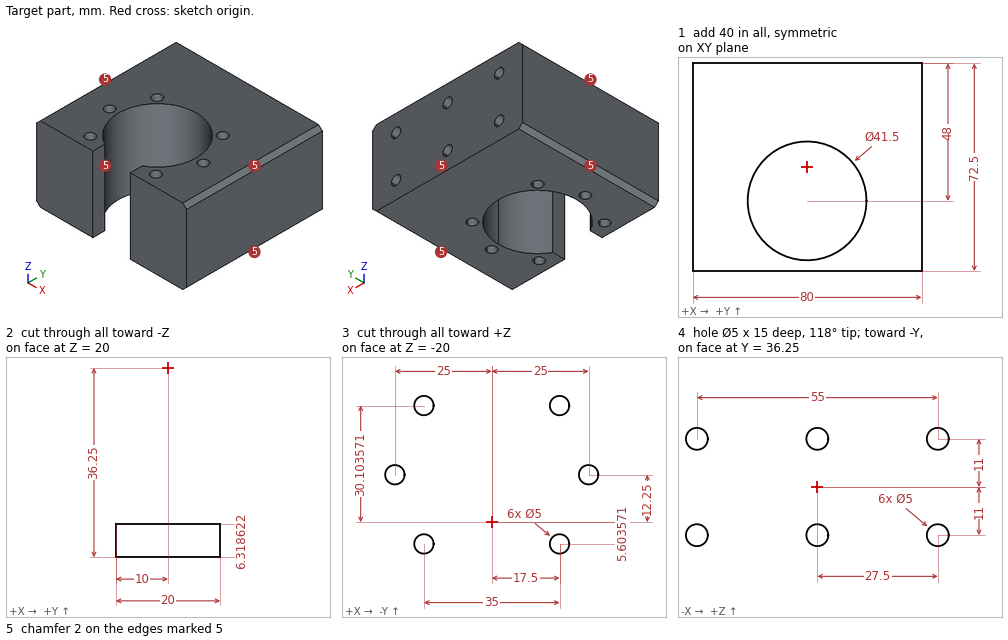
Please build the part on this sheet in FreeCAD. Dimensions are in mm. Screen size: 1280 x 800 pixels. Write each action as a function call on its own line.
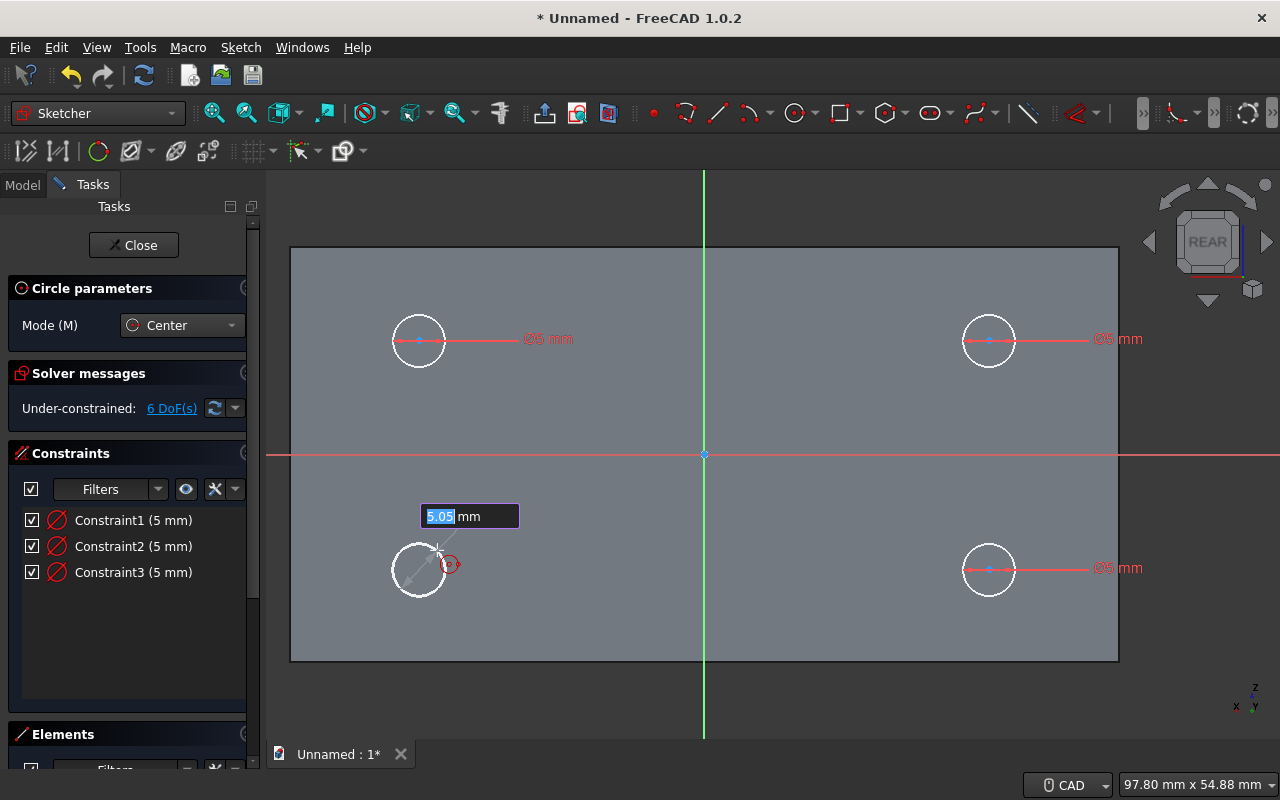
text(5)
key(Return)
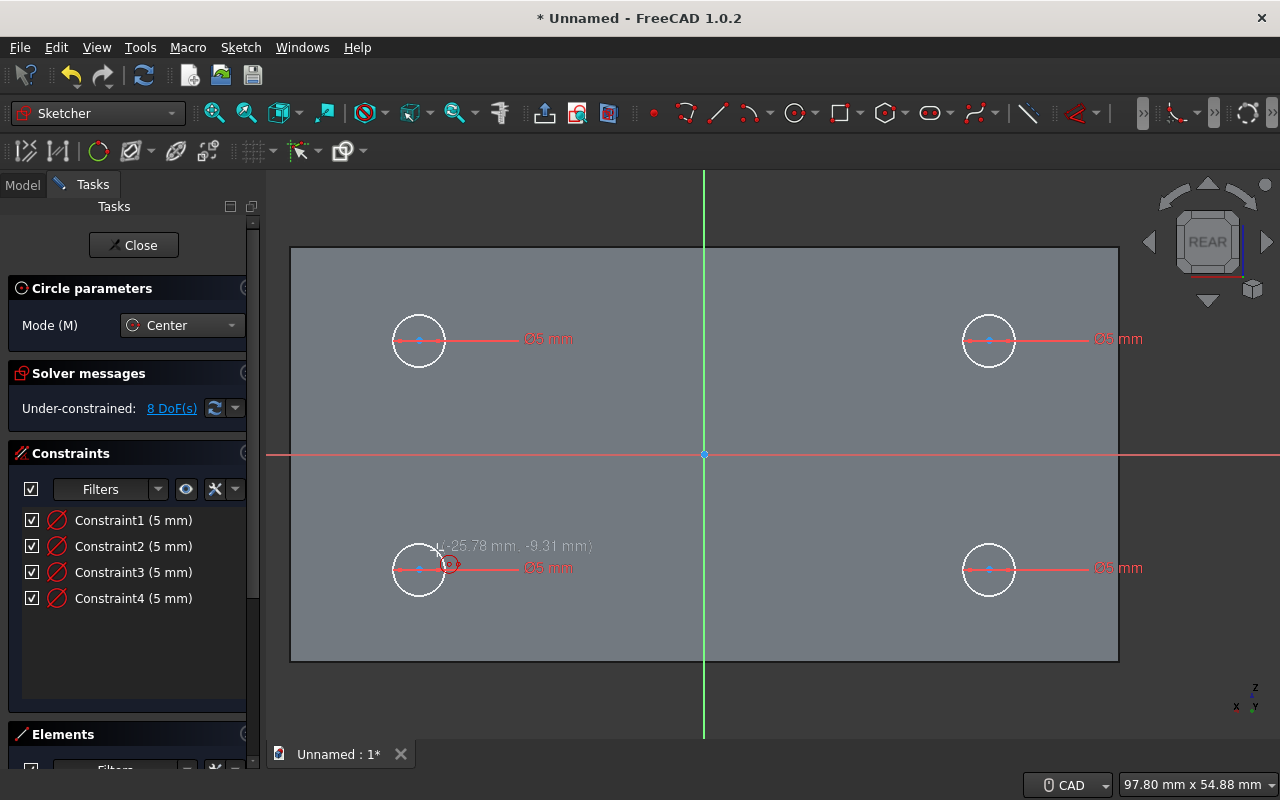
click(704, 569)
move(723, 550)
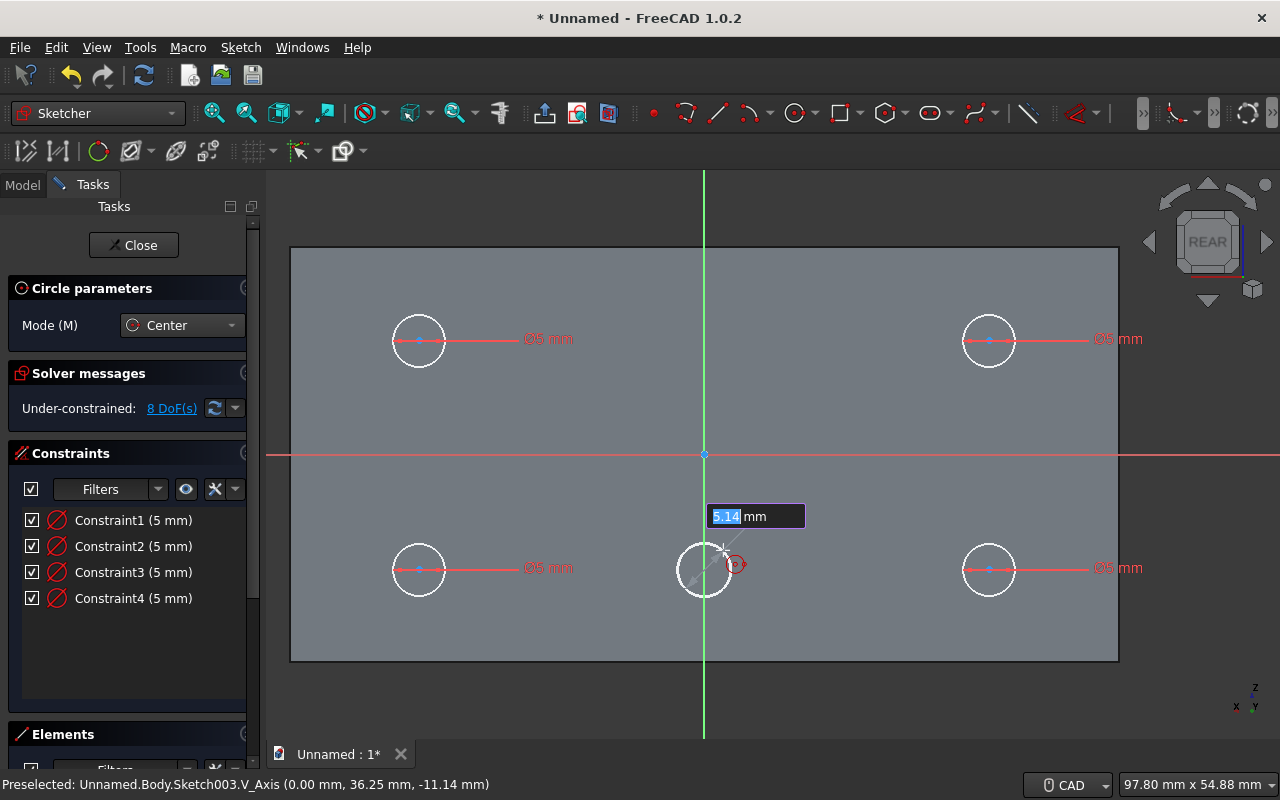
text(5)
key(Return)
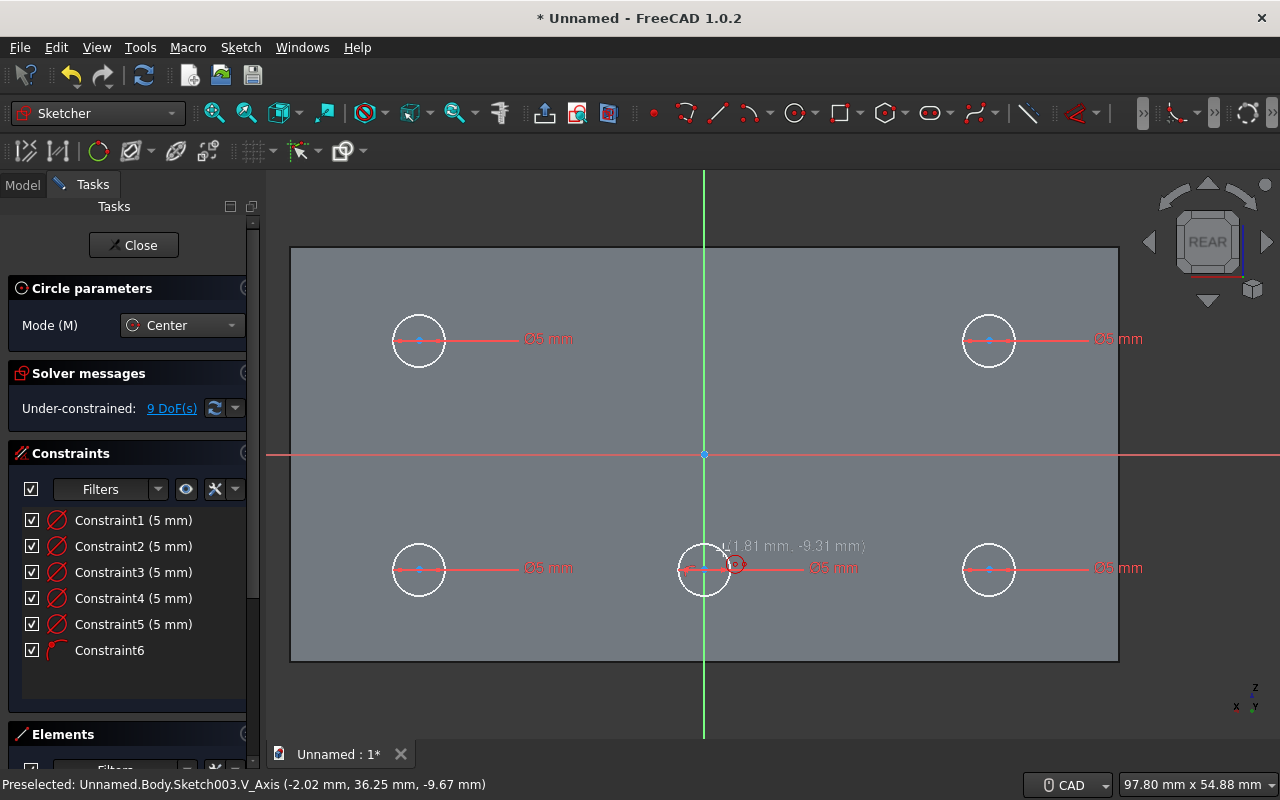
click(704, 340)
move(723, 322)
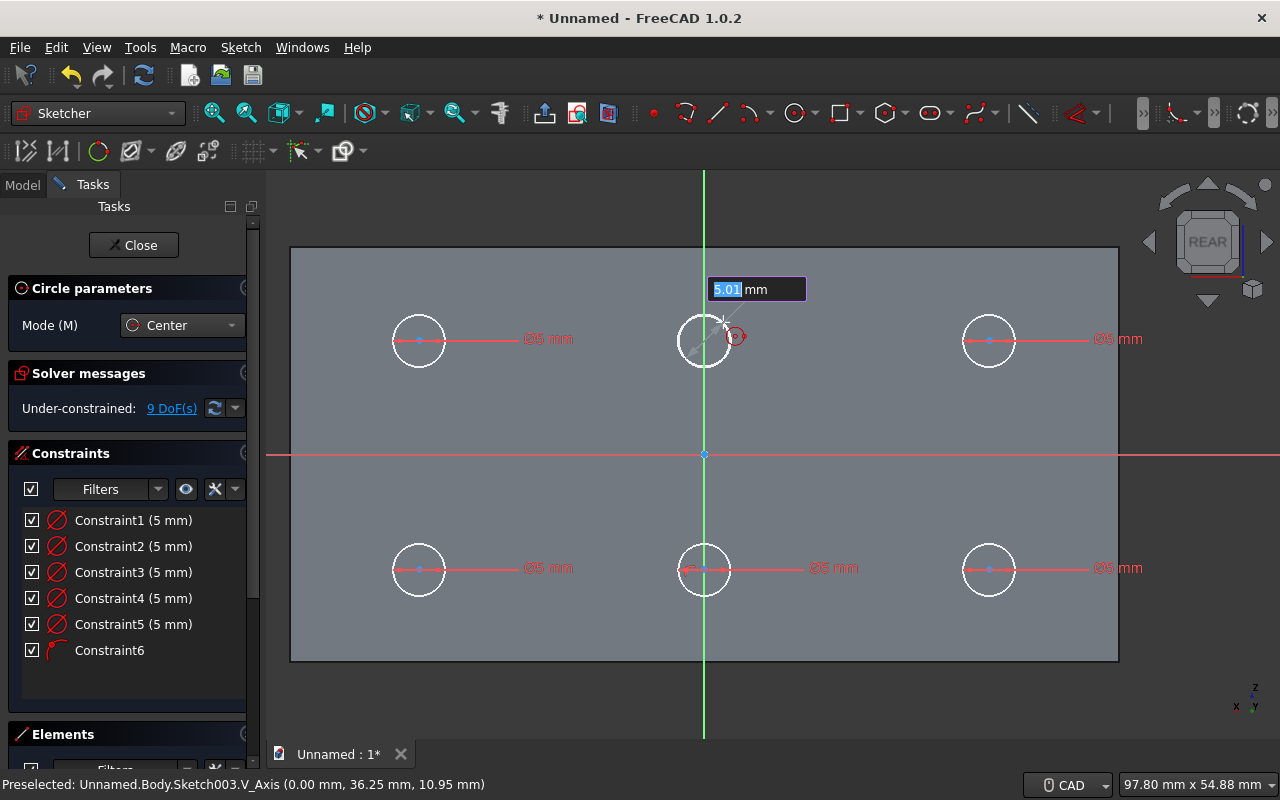
text(5)
key(Return)
key(Escape)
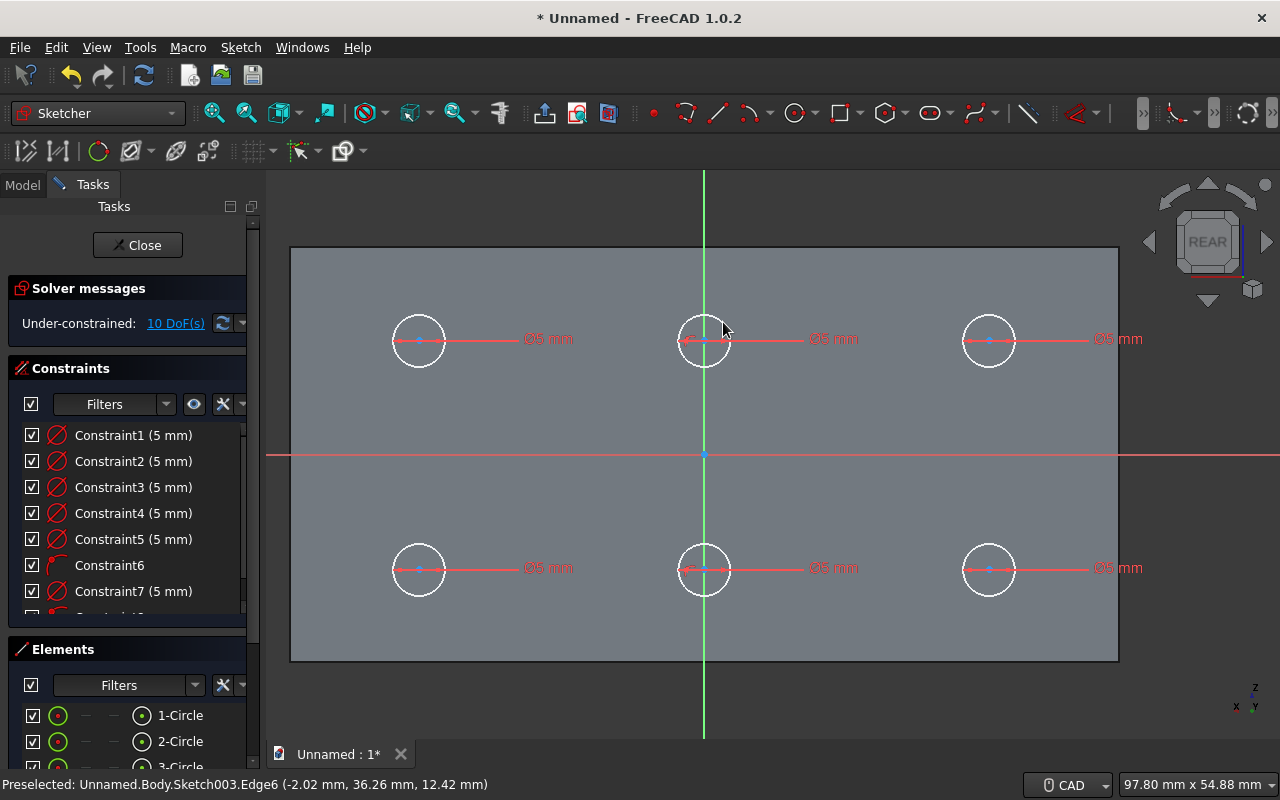
click(989, 570)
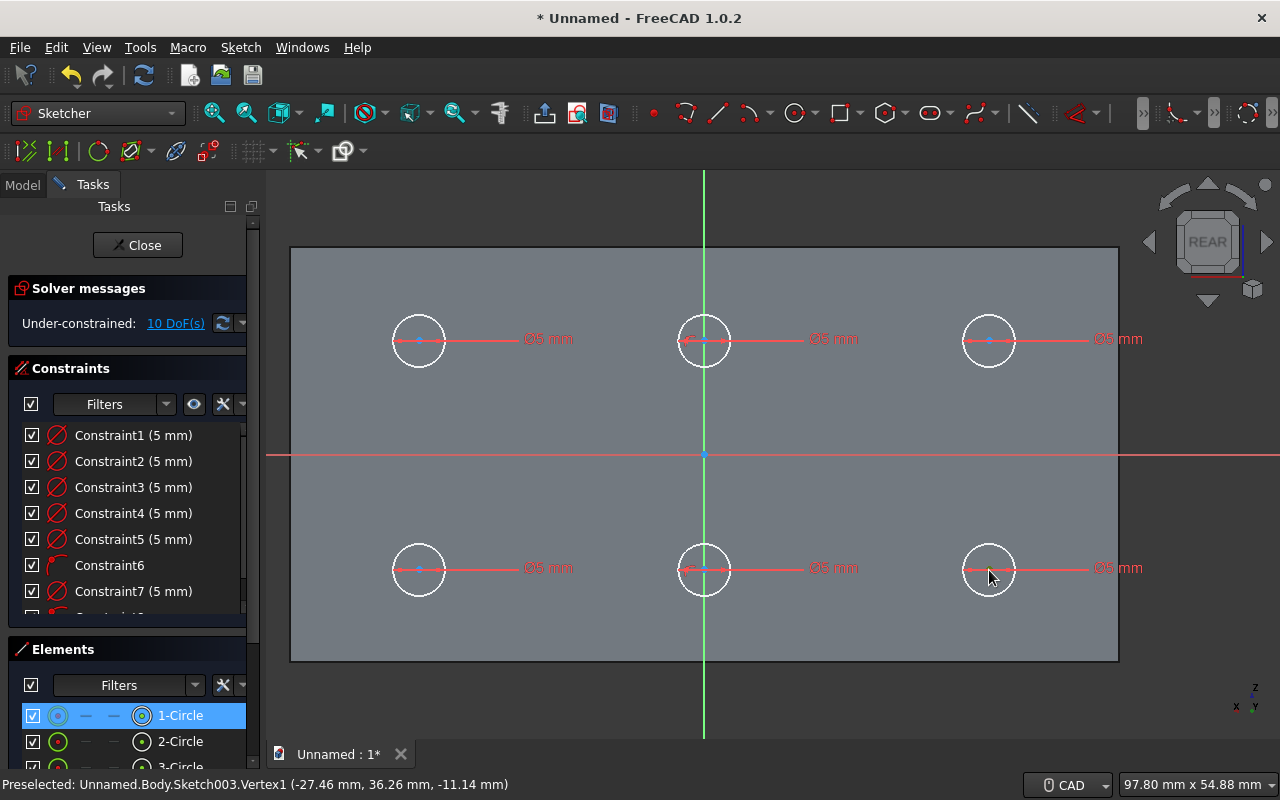
click(989, 341)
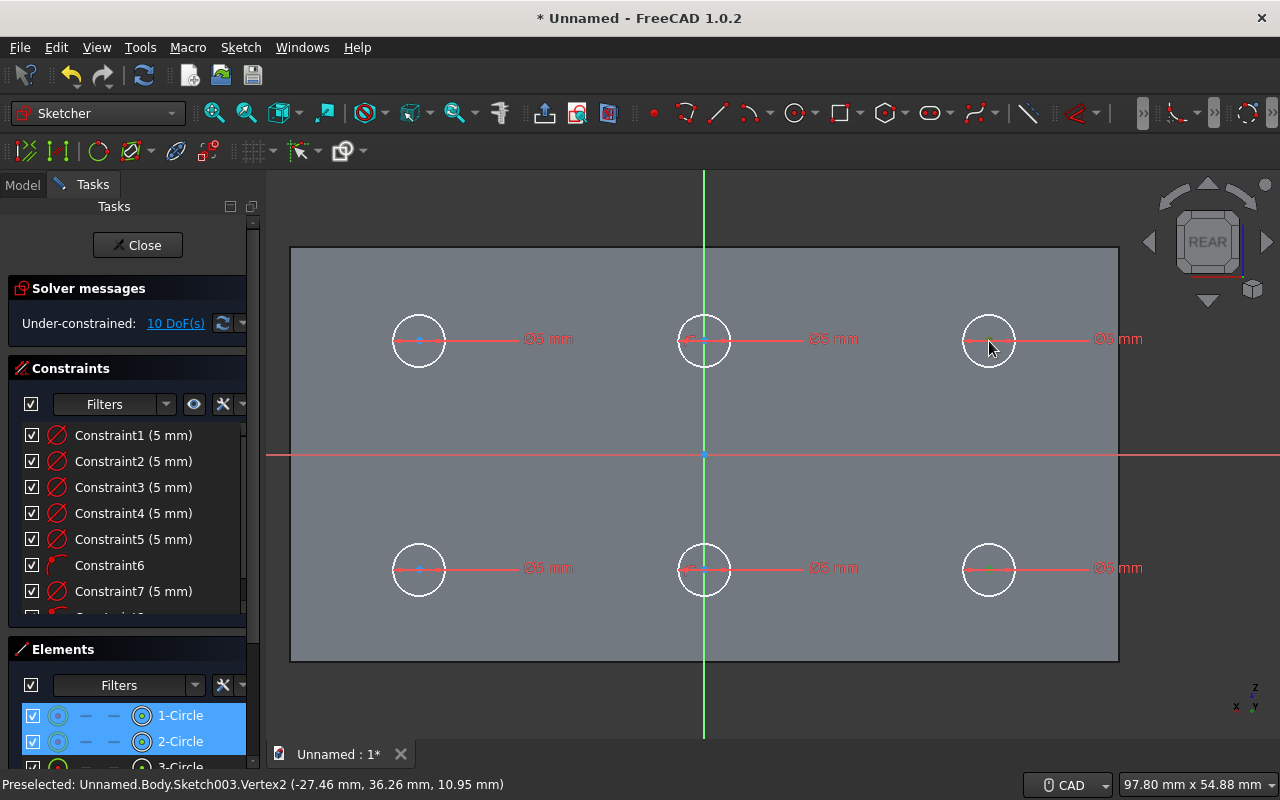
key(v)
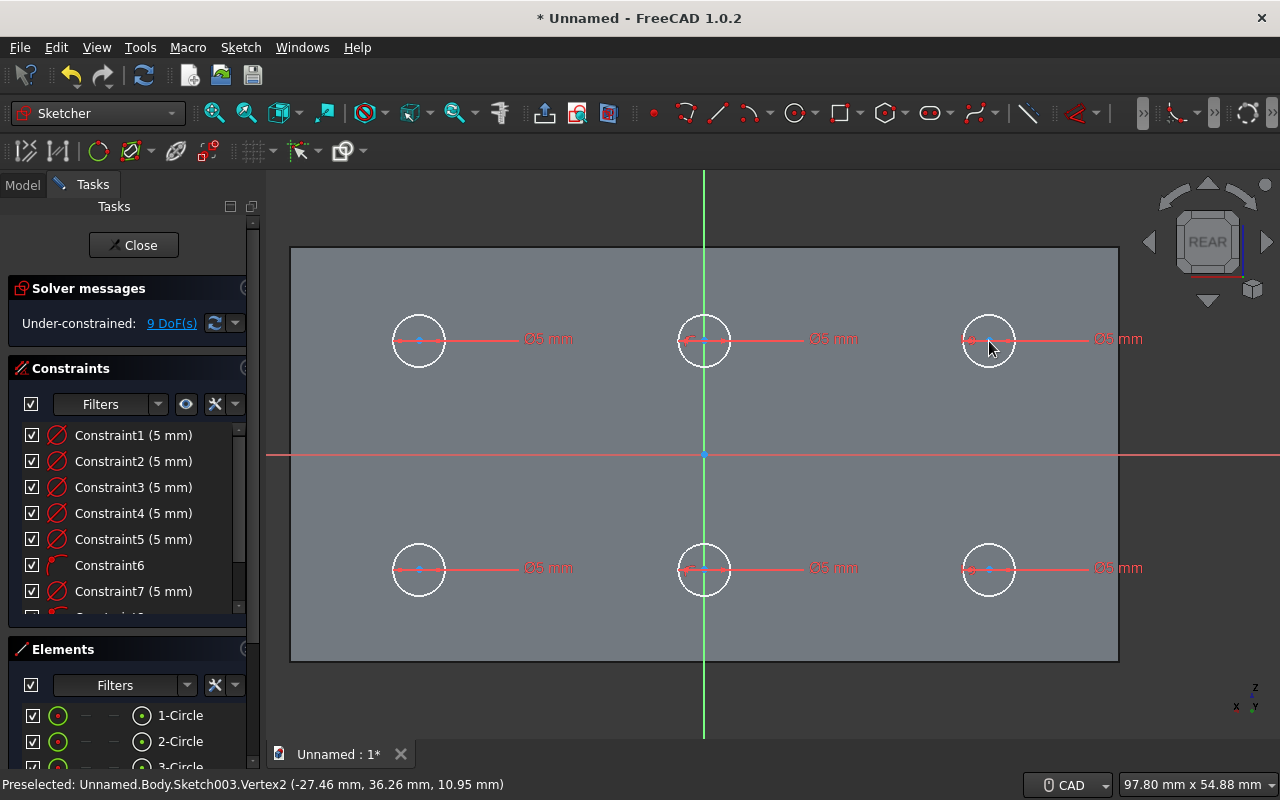
click(989, 341)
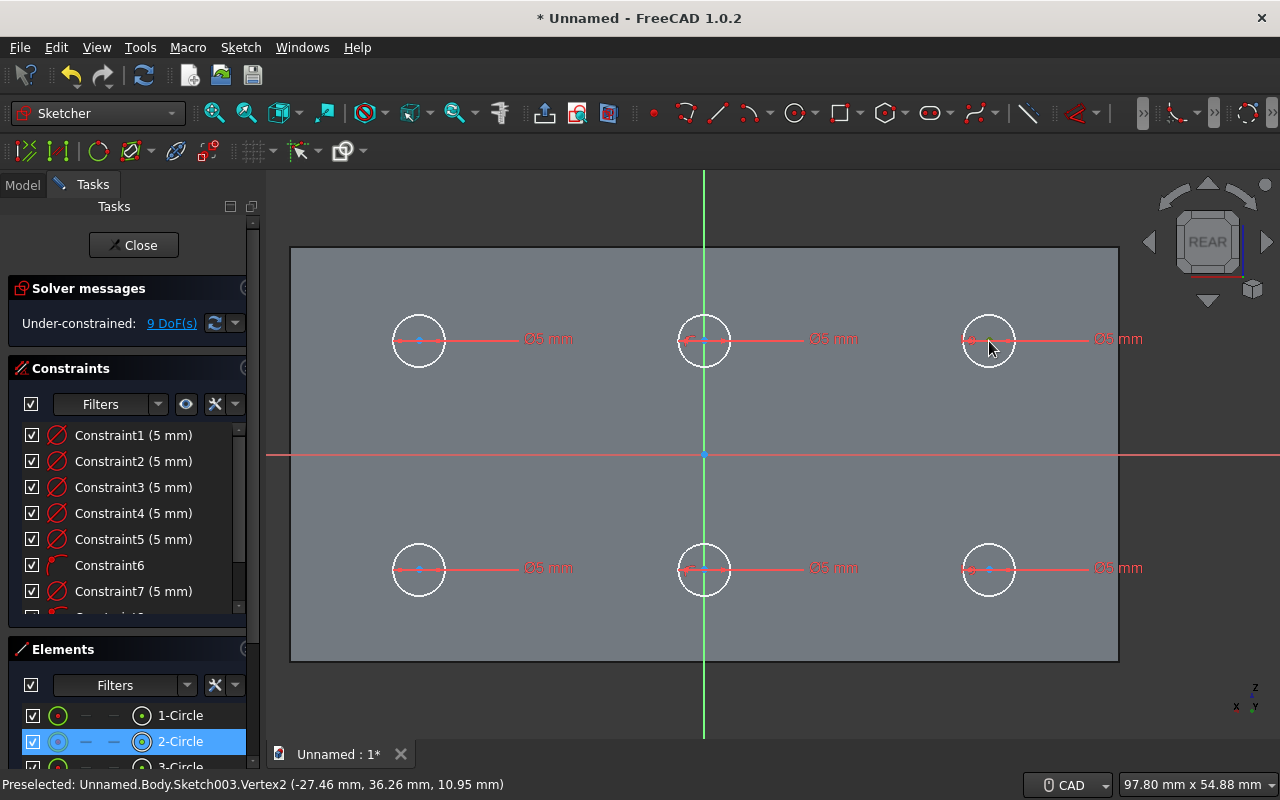
click(419, 341)